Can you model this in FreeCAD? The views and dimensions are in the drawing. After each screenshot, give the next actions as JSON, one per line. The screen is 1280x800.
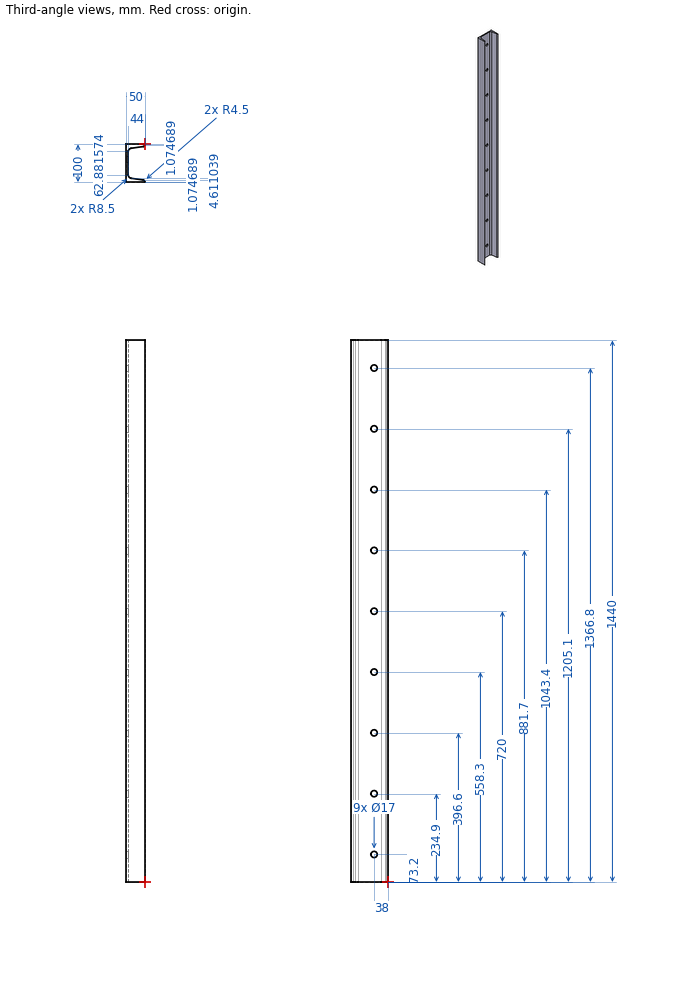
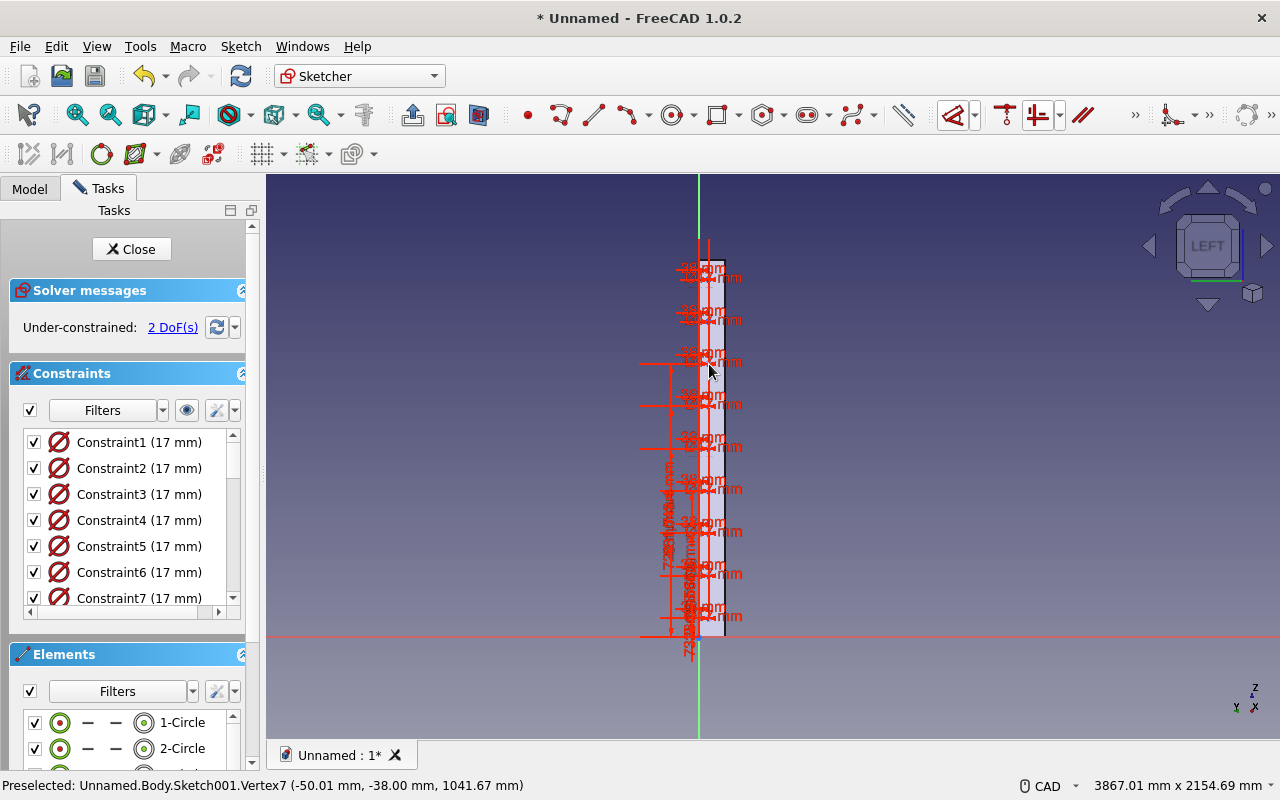
{"action": "left_click", "coordinate": [709, 322]}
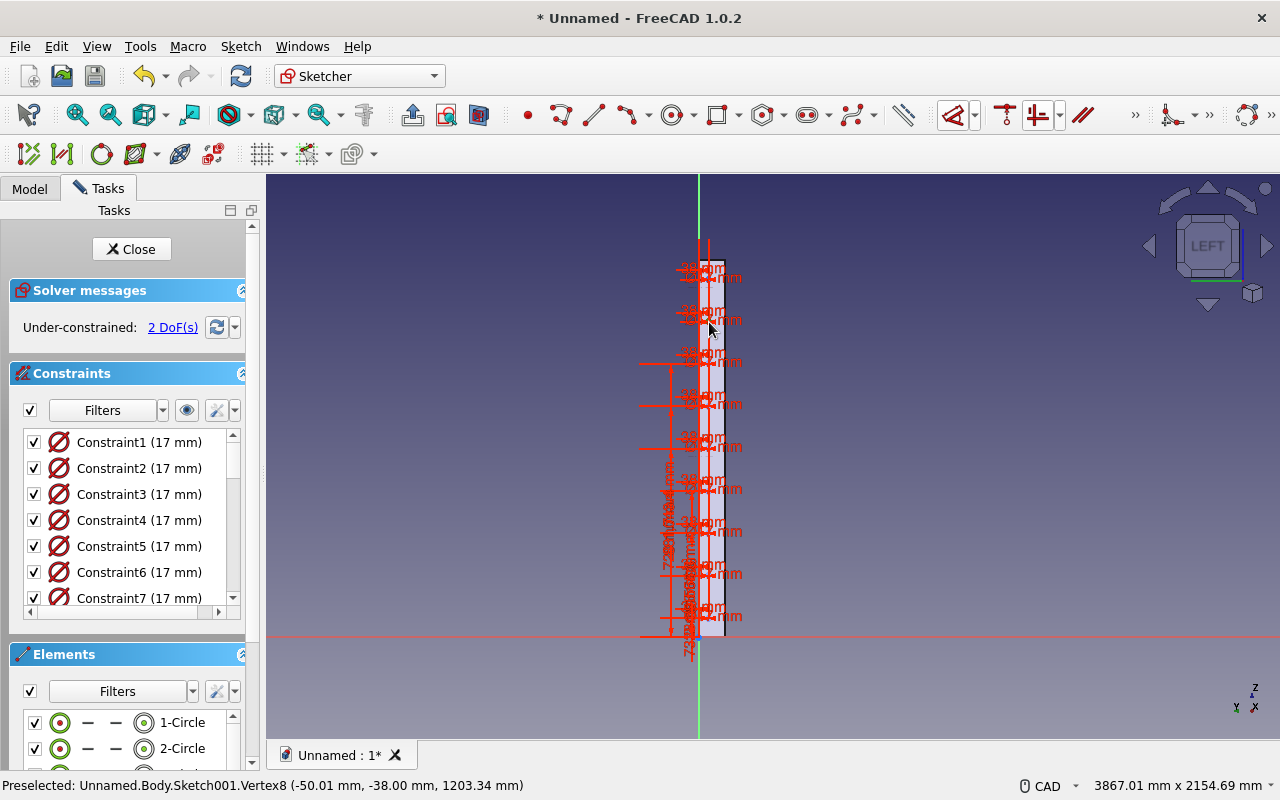
{"action": "key", "text": "i"}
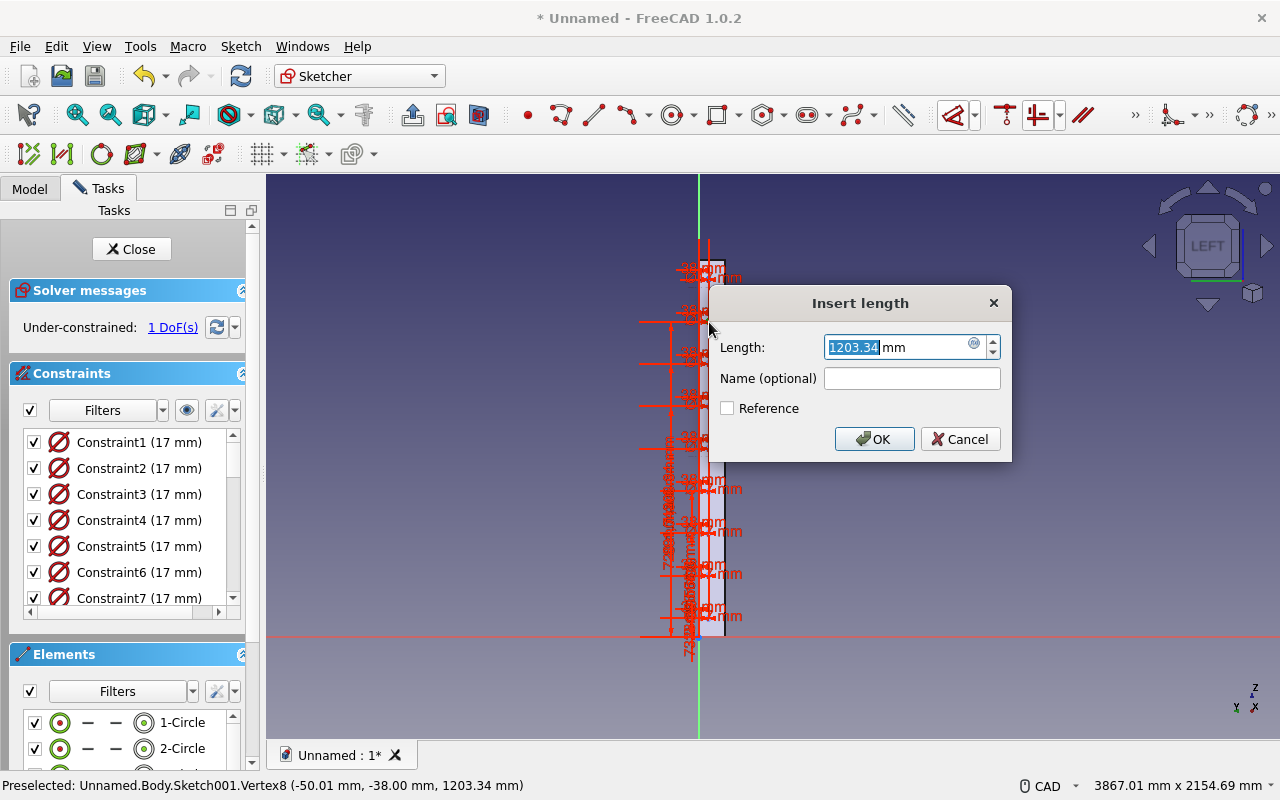
{"action": "type", "text": "1205.1"}
{"action": "key", "text": "Return"}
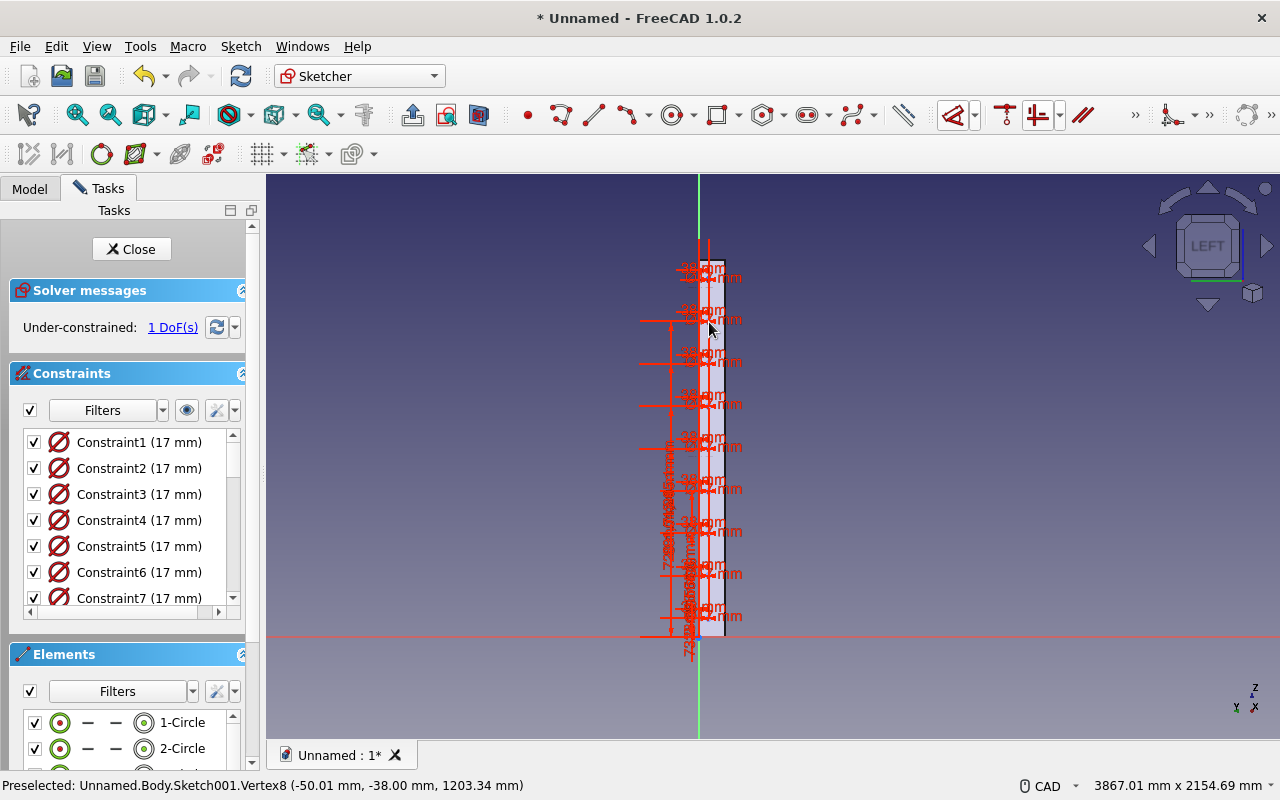
{"action": "left_click", "coordinate": [709, 280]}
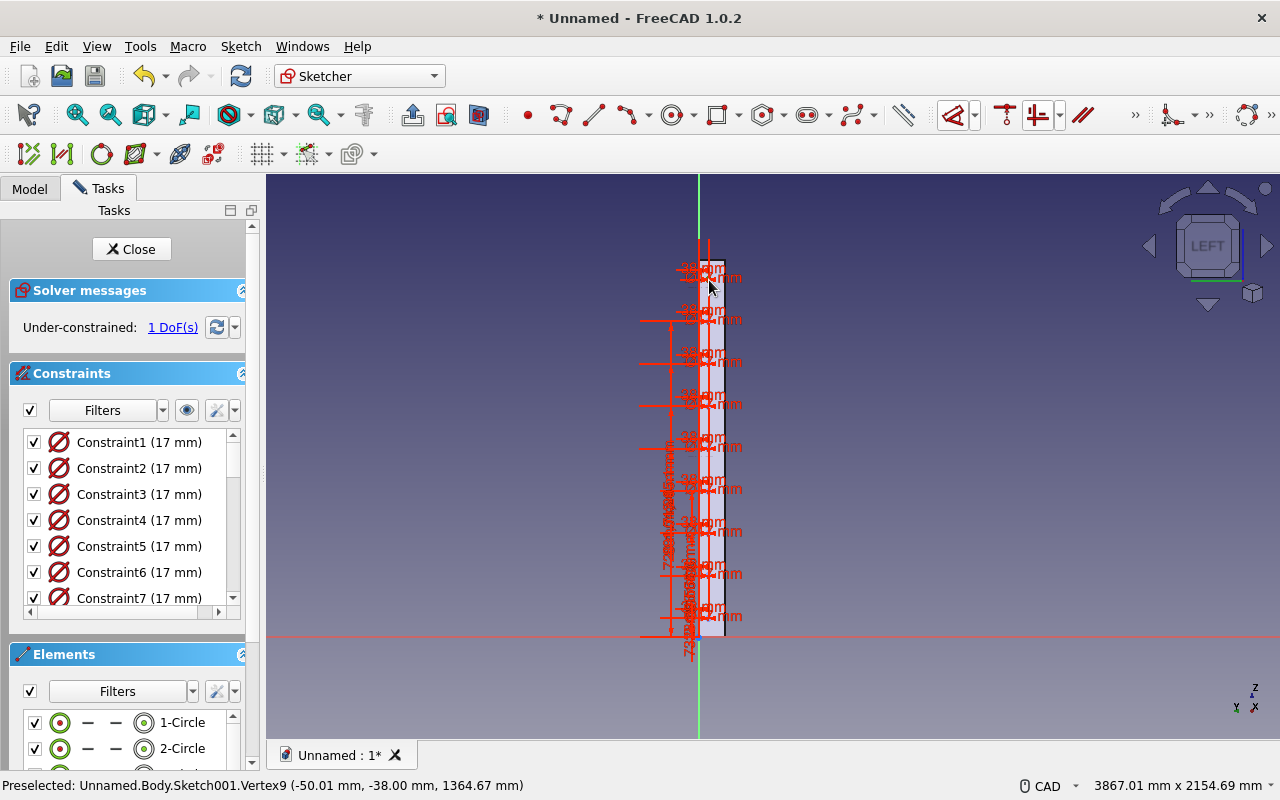
{"action": "left_click", "coordinate": [974, 116]}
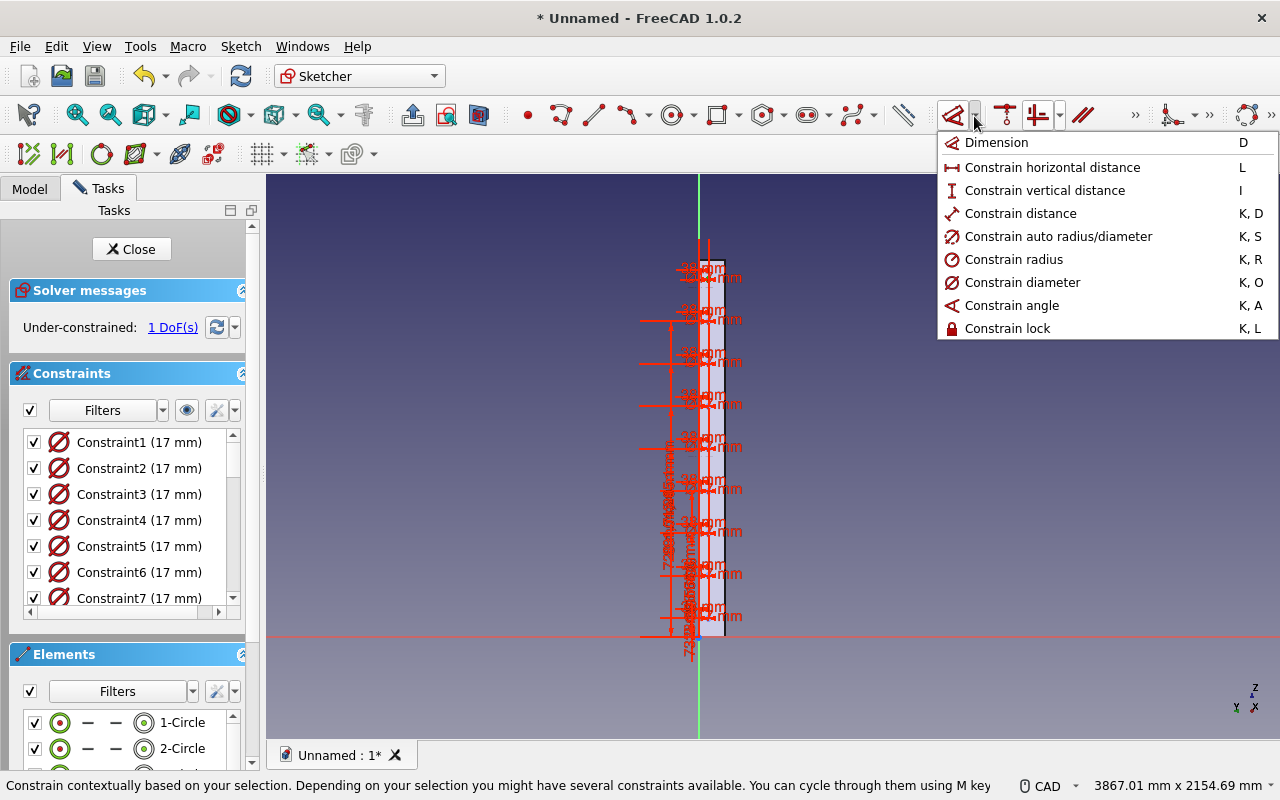
{"action": "left_click", "coordinate": [1108, 190]}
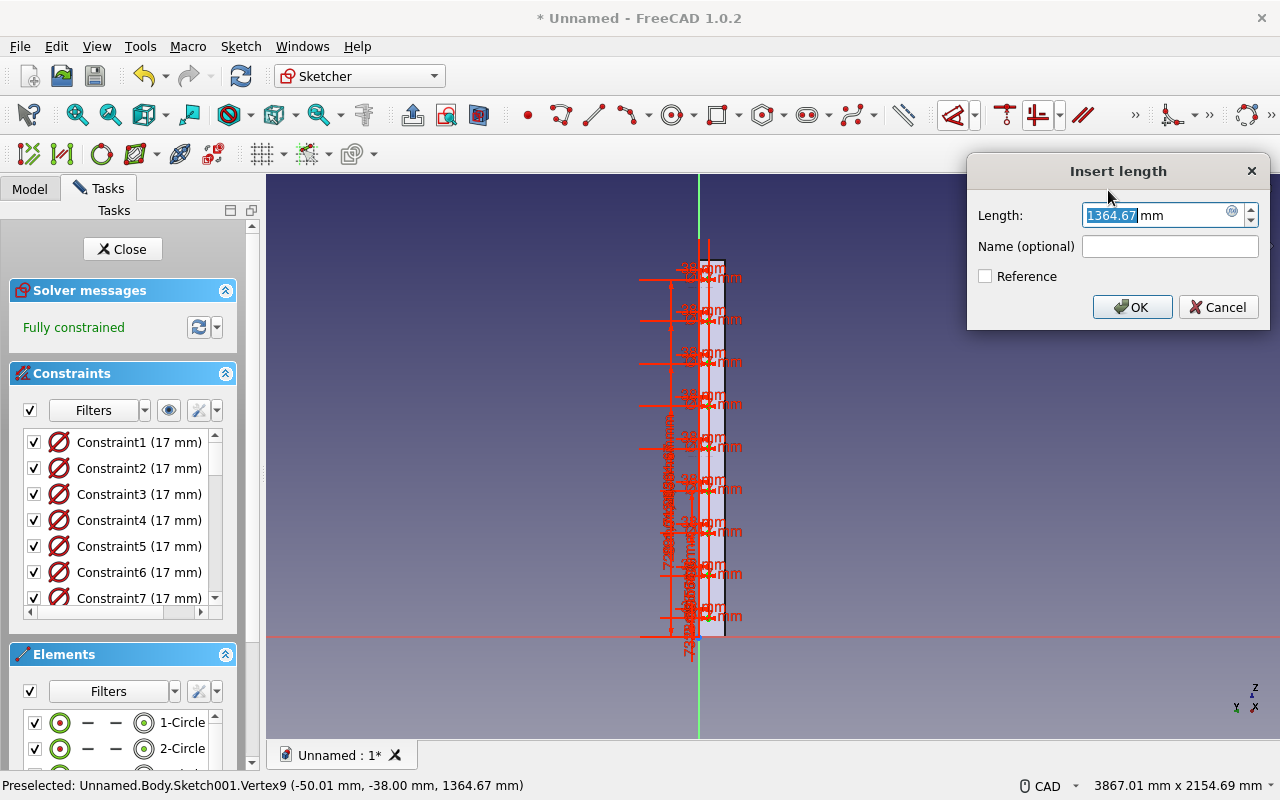
{"action": "type", "text": "1366.8"}
{"action": "key", "text": "Return"}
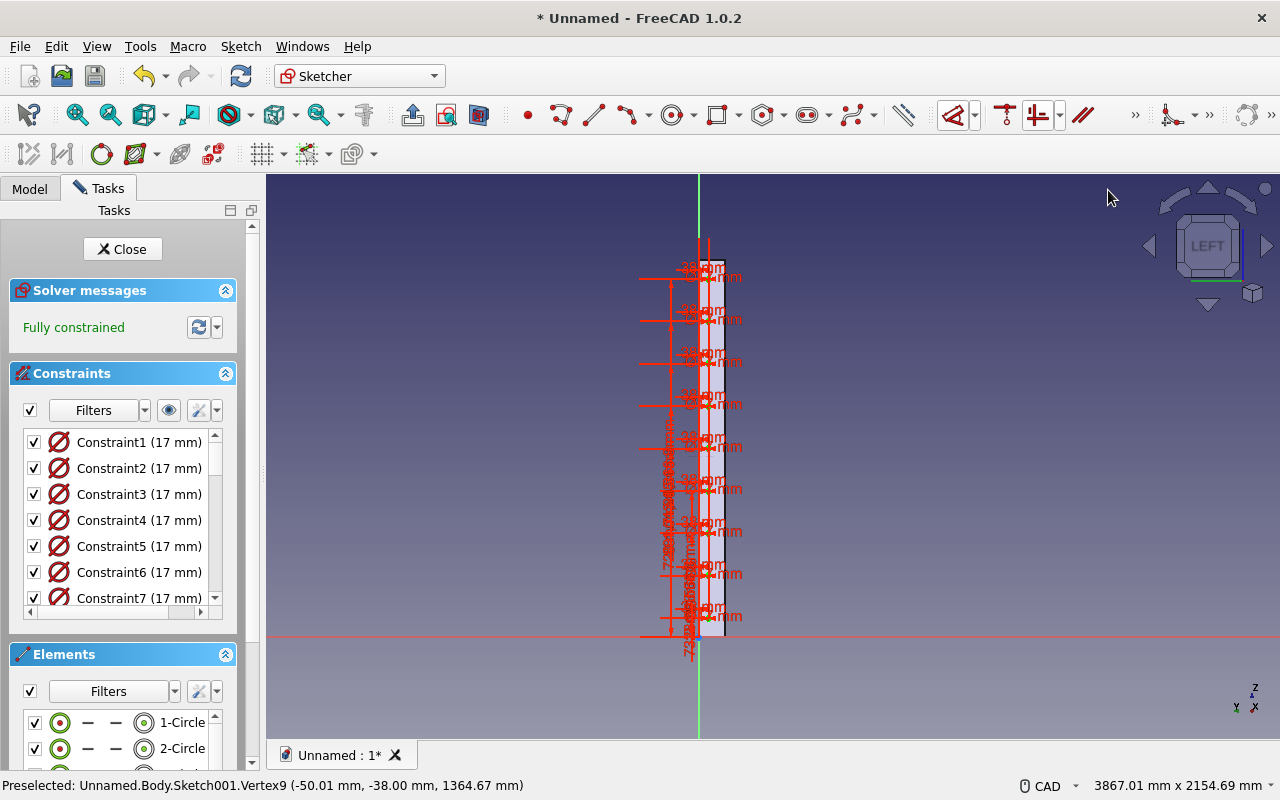
{"action": "left_click", "coordinate": [123, 249]}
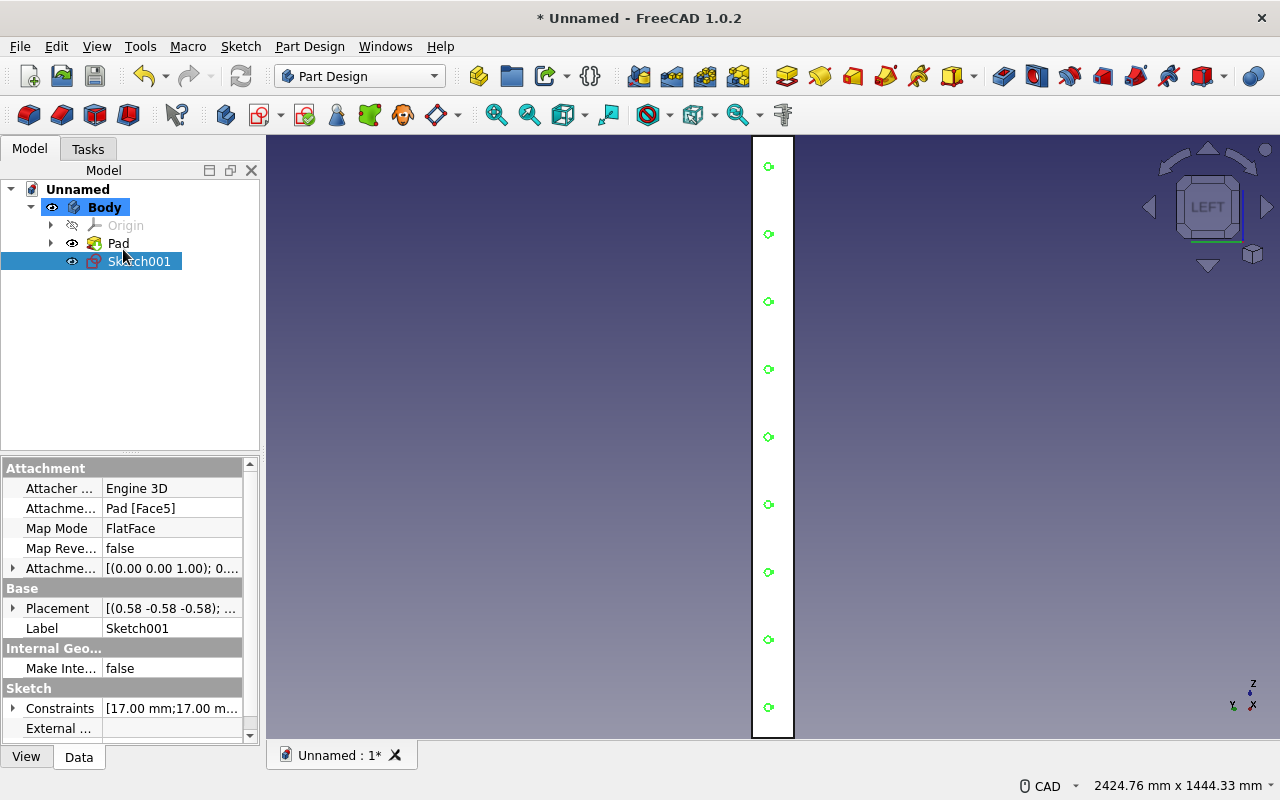
{"action": "left_click", "coordinate": [1004, 76]}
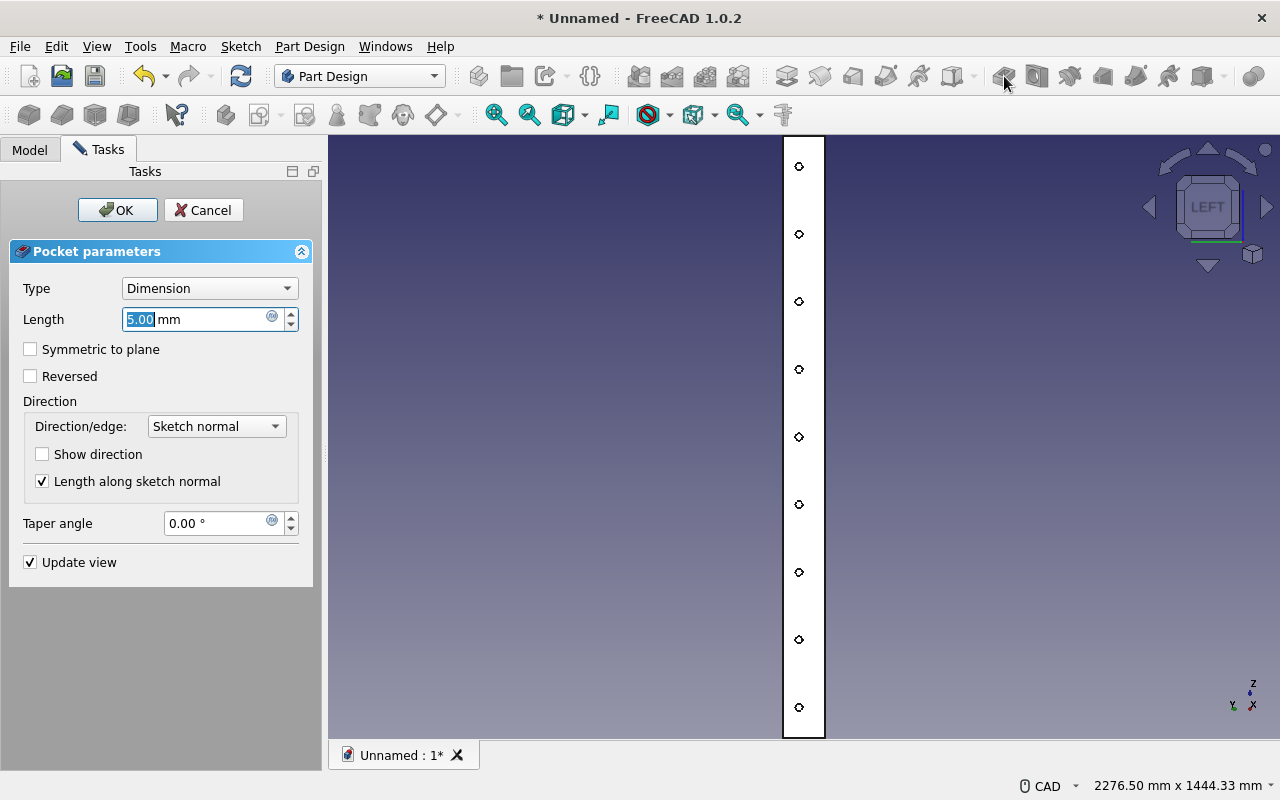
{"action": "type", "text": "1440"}
{"action": "key", "text": "Tab"}